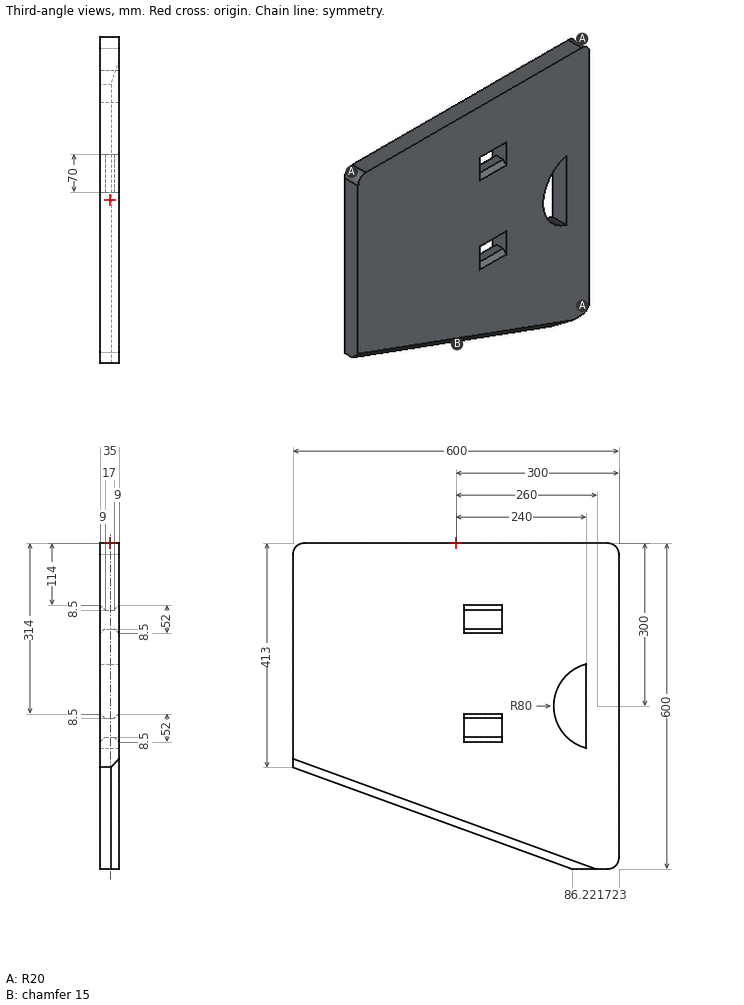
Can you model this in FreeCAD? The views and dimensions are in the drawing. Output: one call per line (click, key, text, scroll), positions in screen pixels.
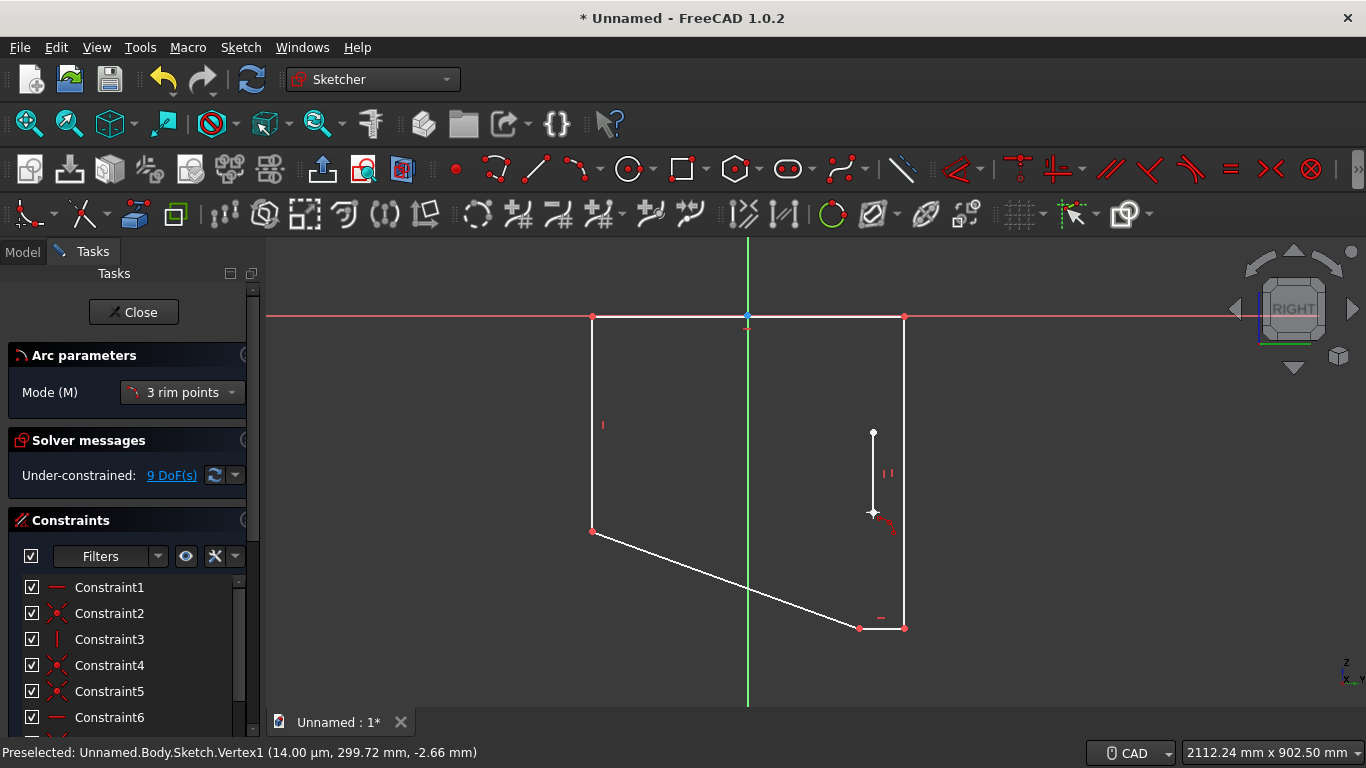
click(873, 513)
click(873, 433)
click(842, 472)
key(Escape)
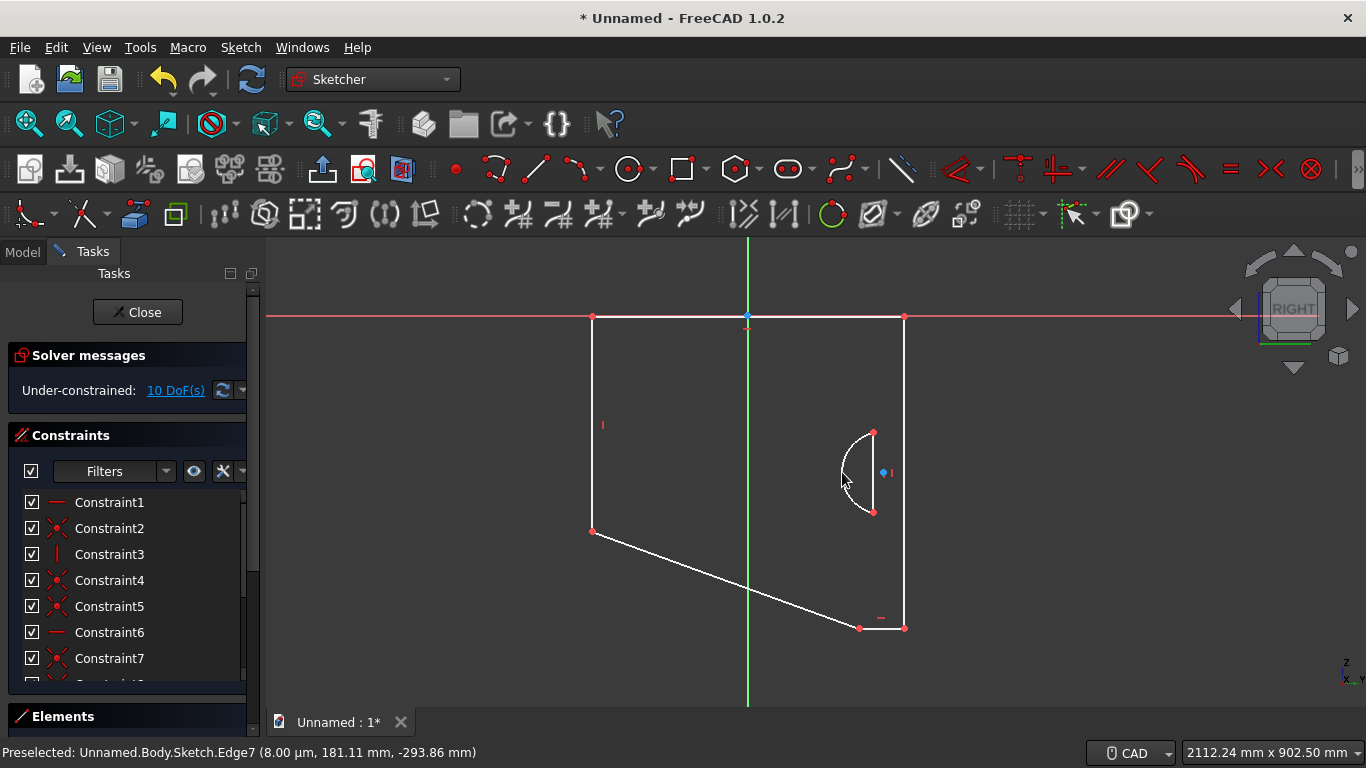
click(848, 452)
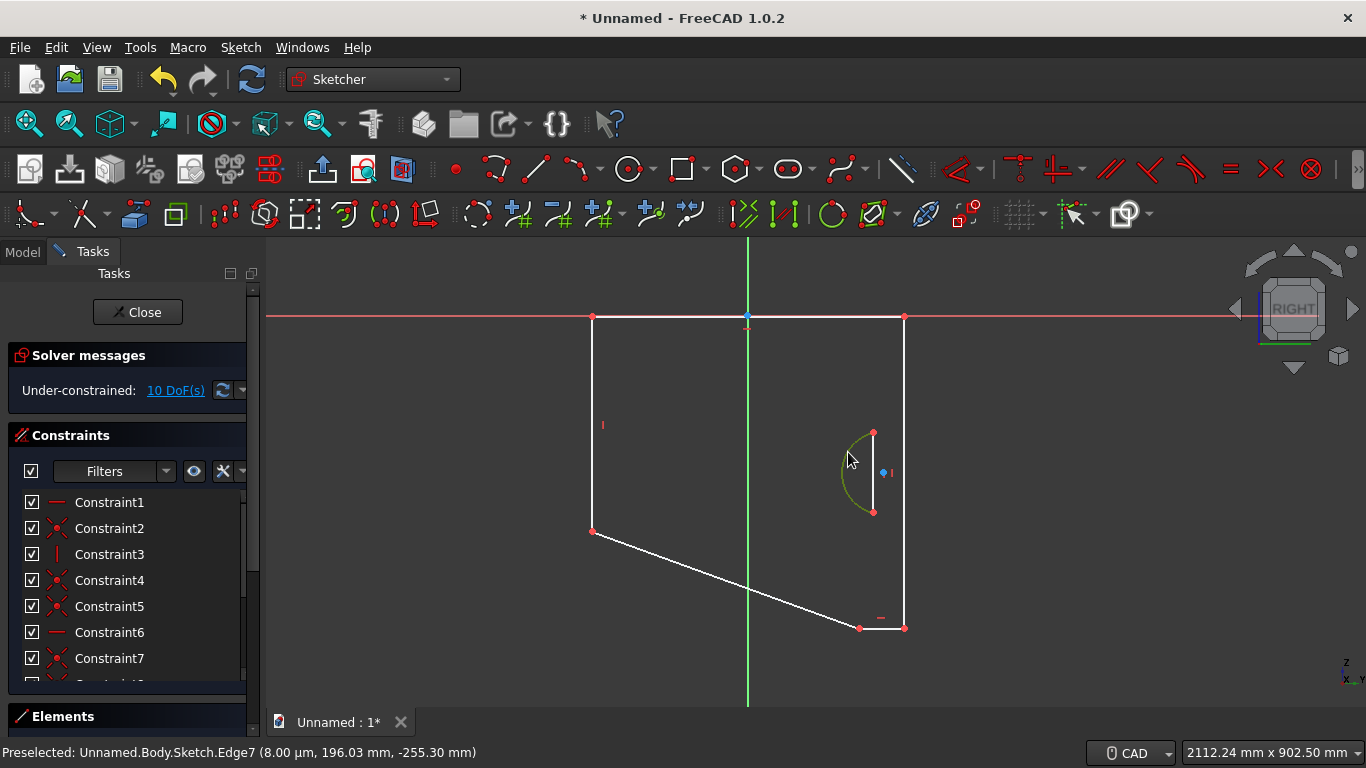
click(982, 170)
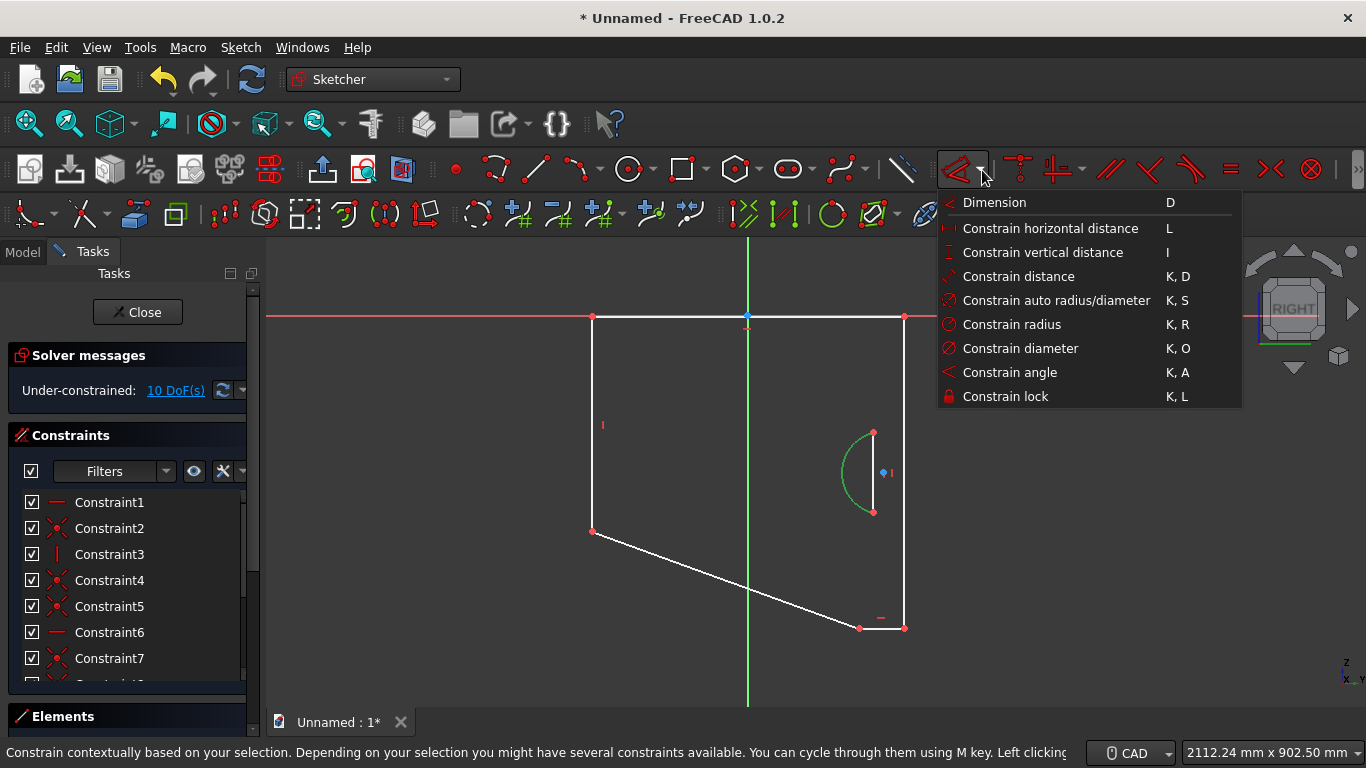
click(1090, 324)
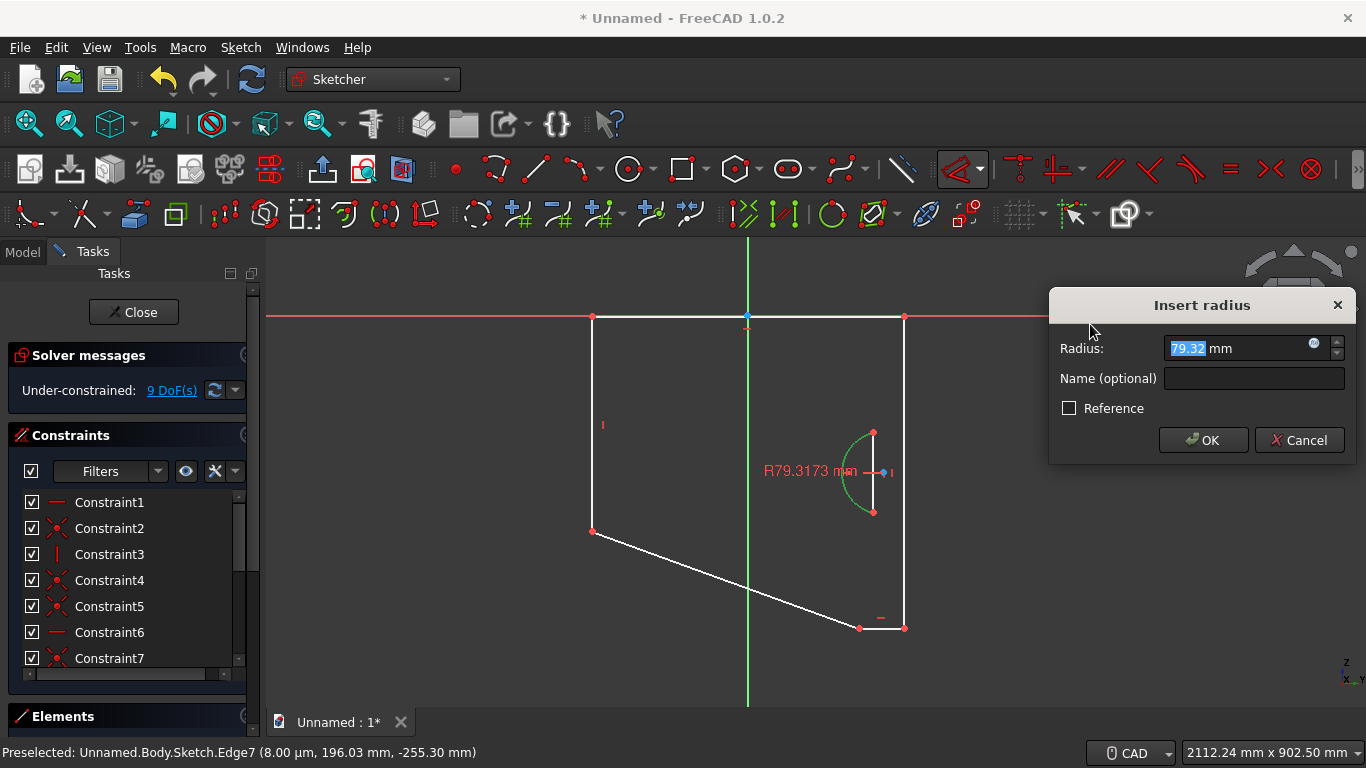
text(80)
key(Return)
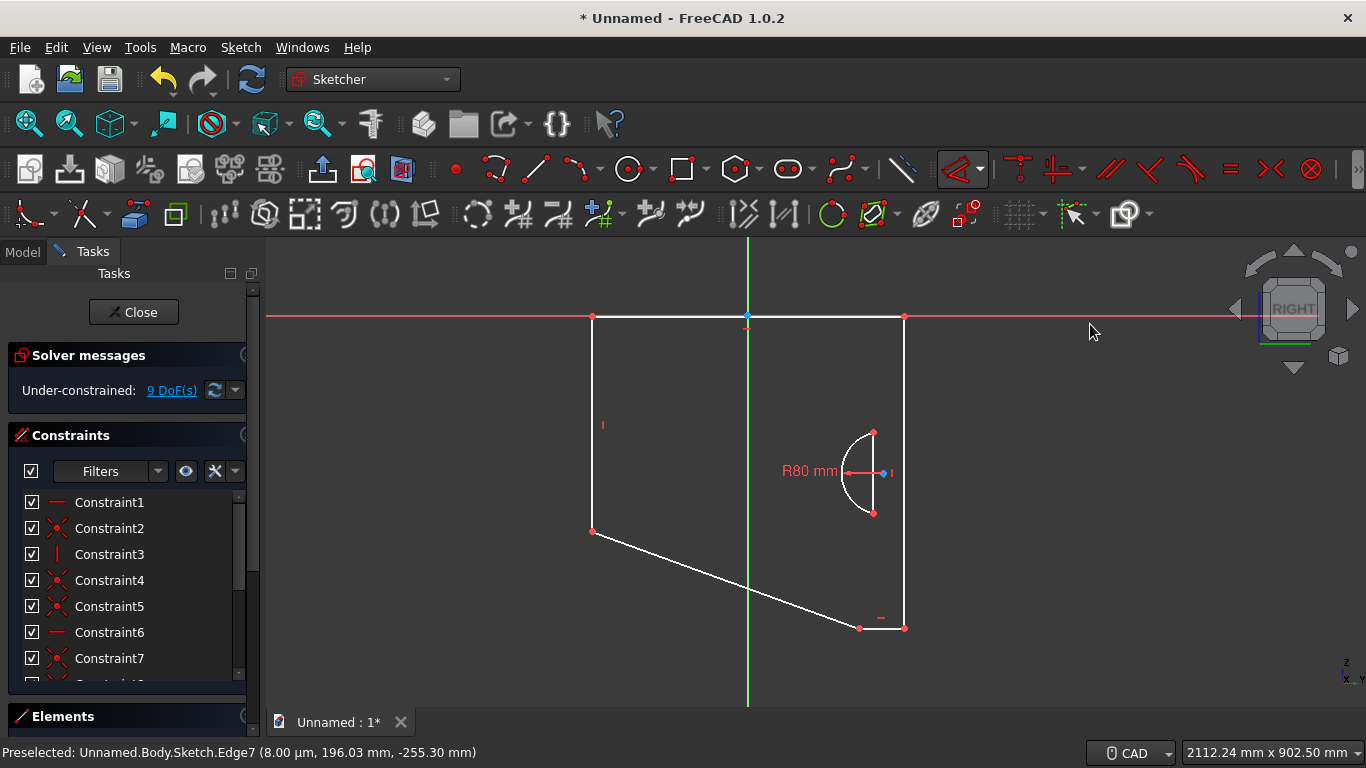
click(904, 317)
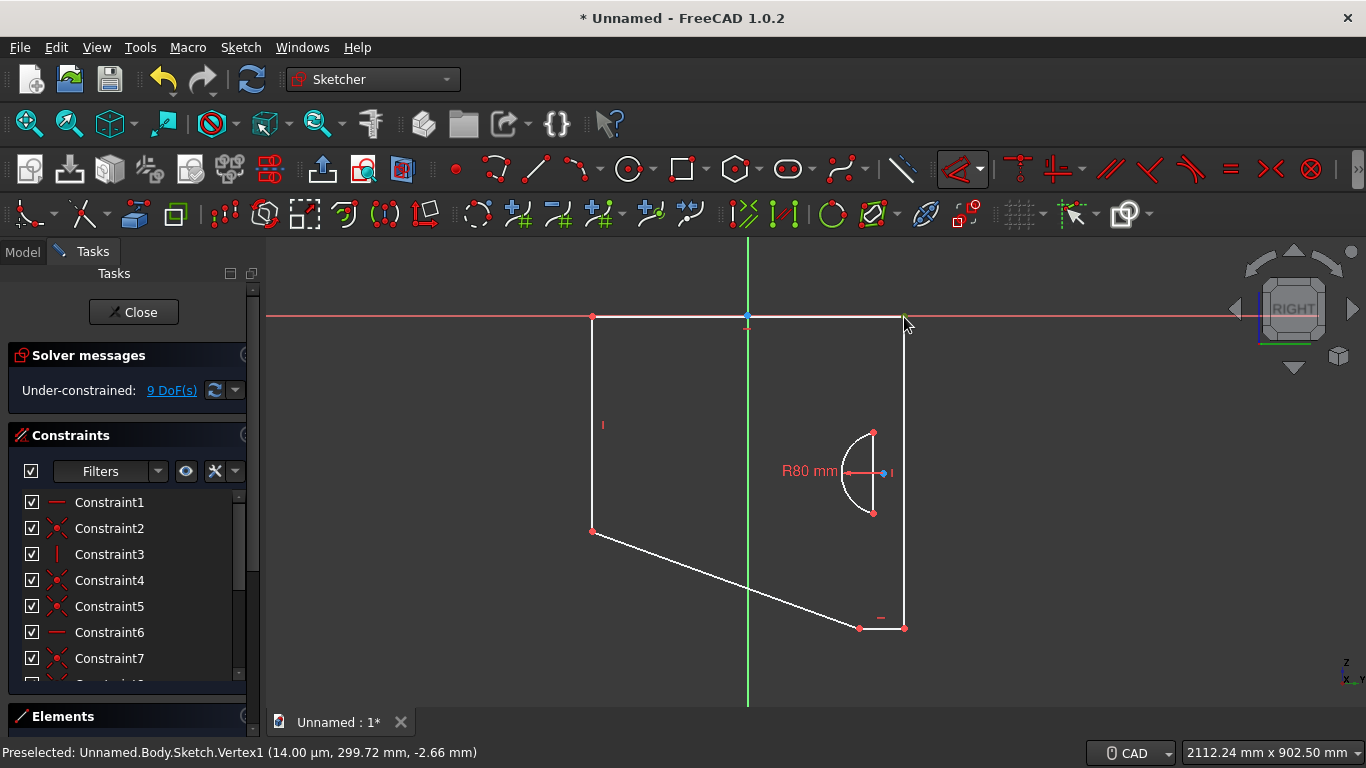
click(359, 316)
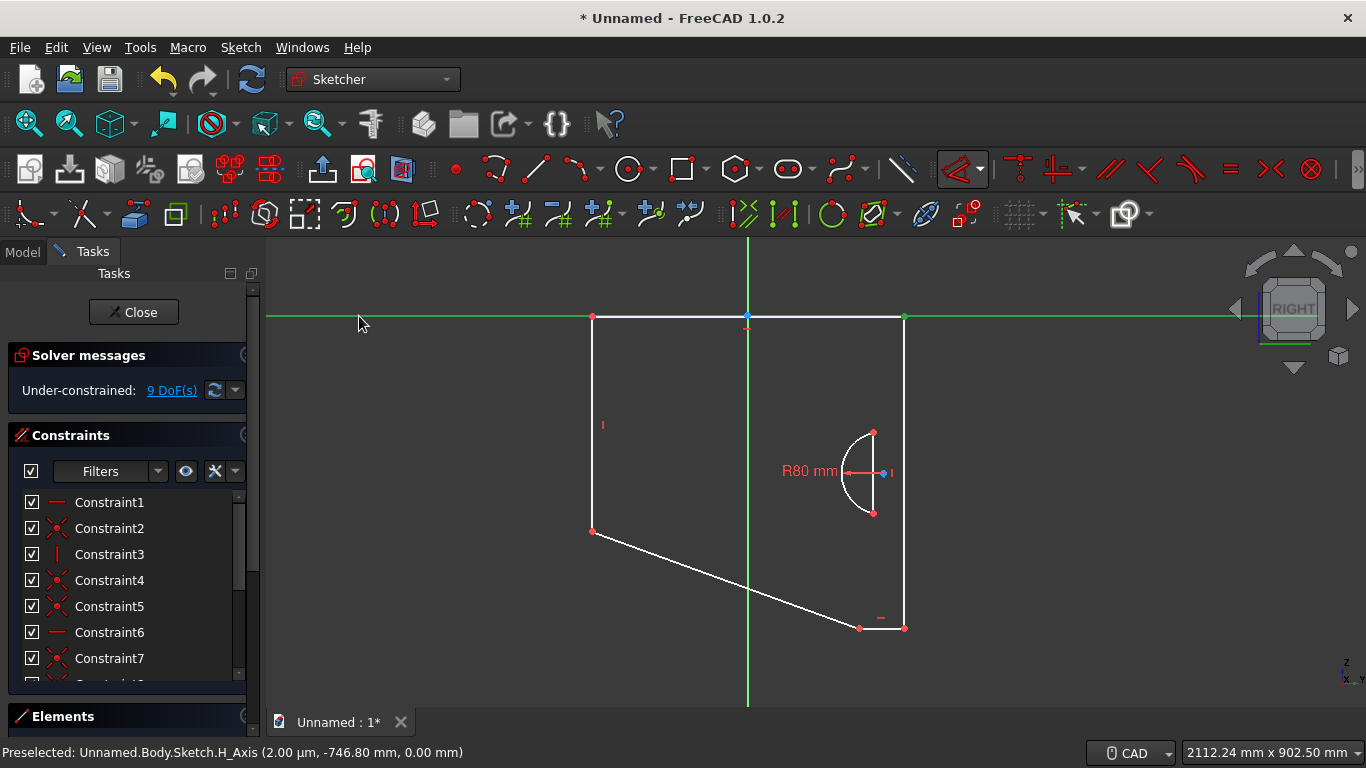
click(1018, 170)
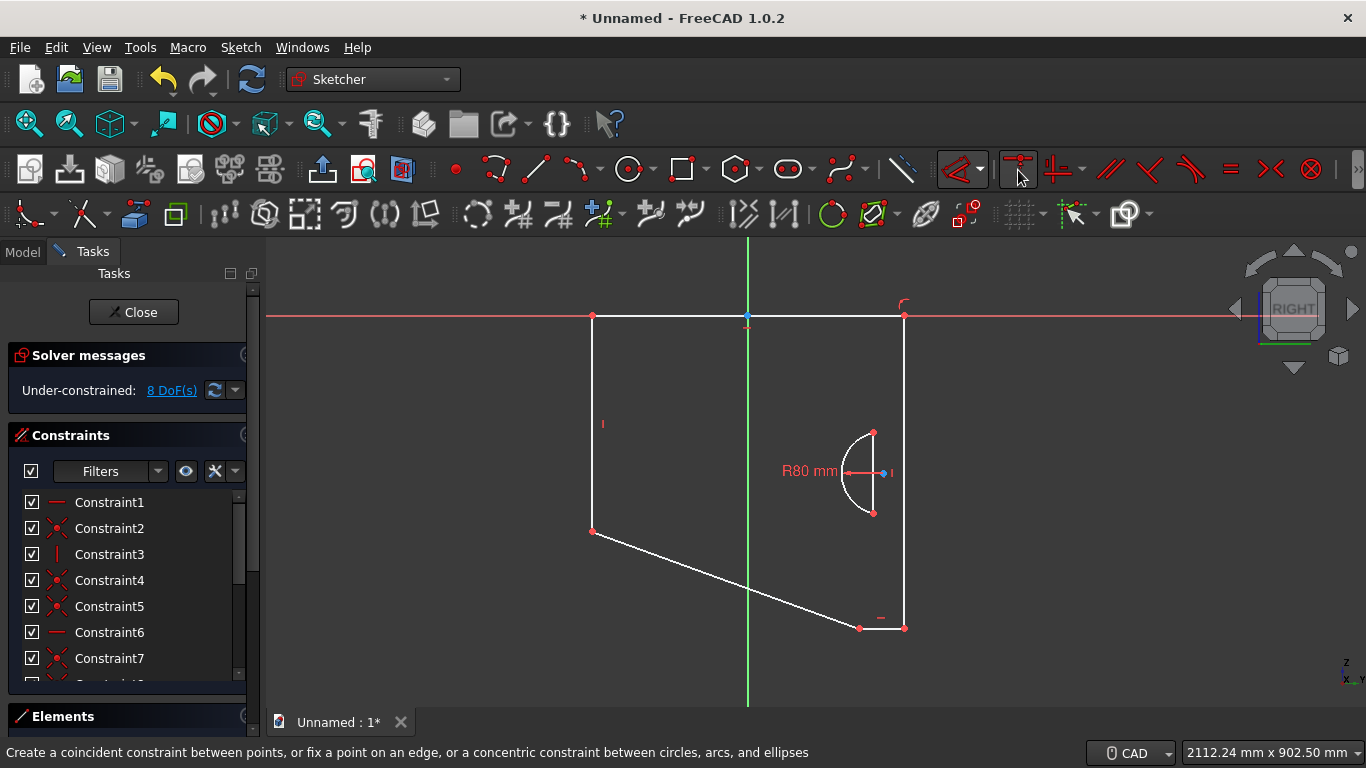
click(810, 316)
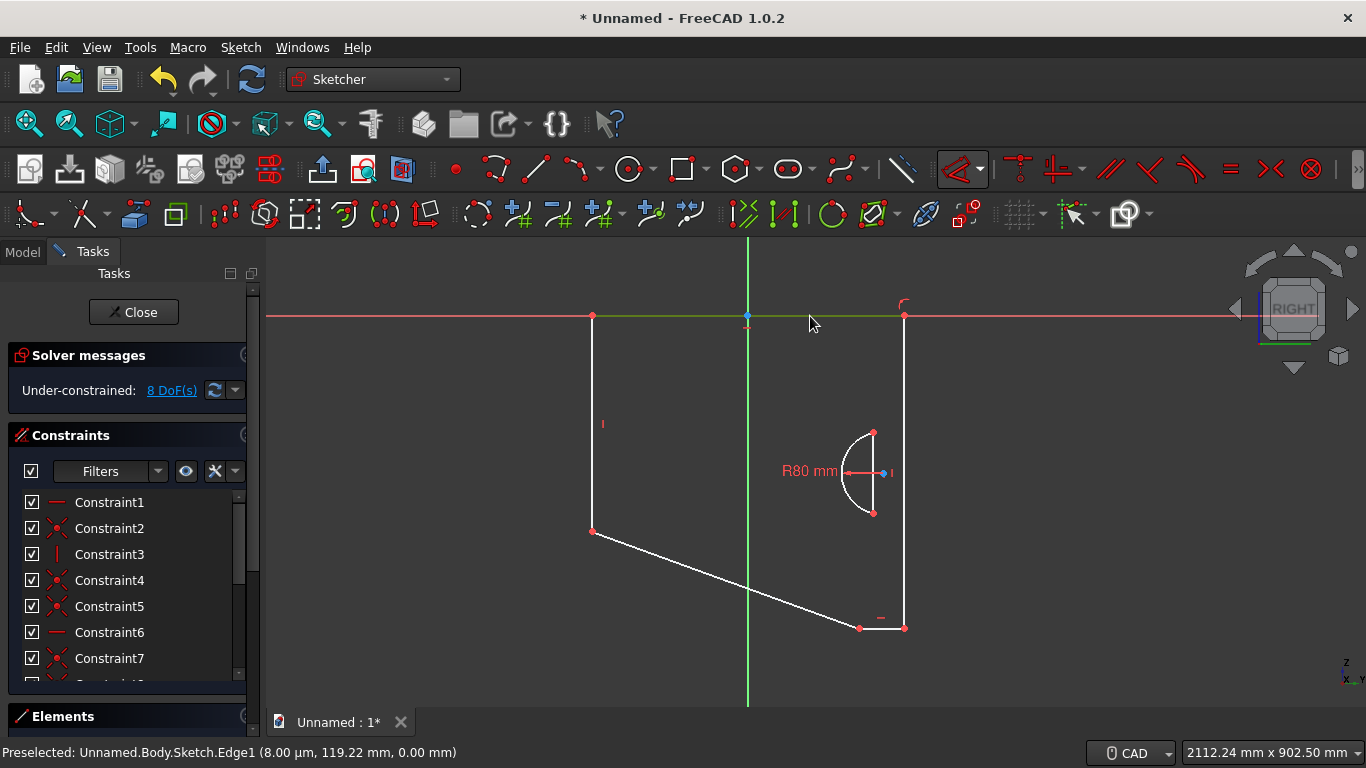
click(982, 170)